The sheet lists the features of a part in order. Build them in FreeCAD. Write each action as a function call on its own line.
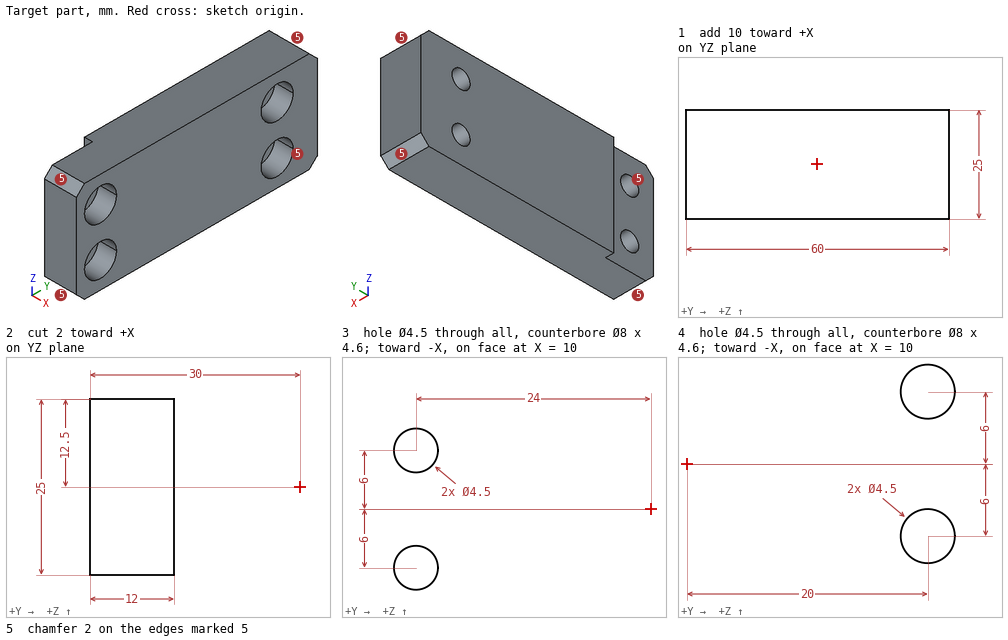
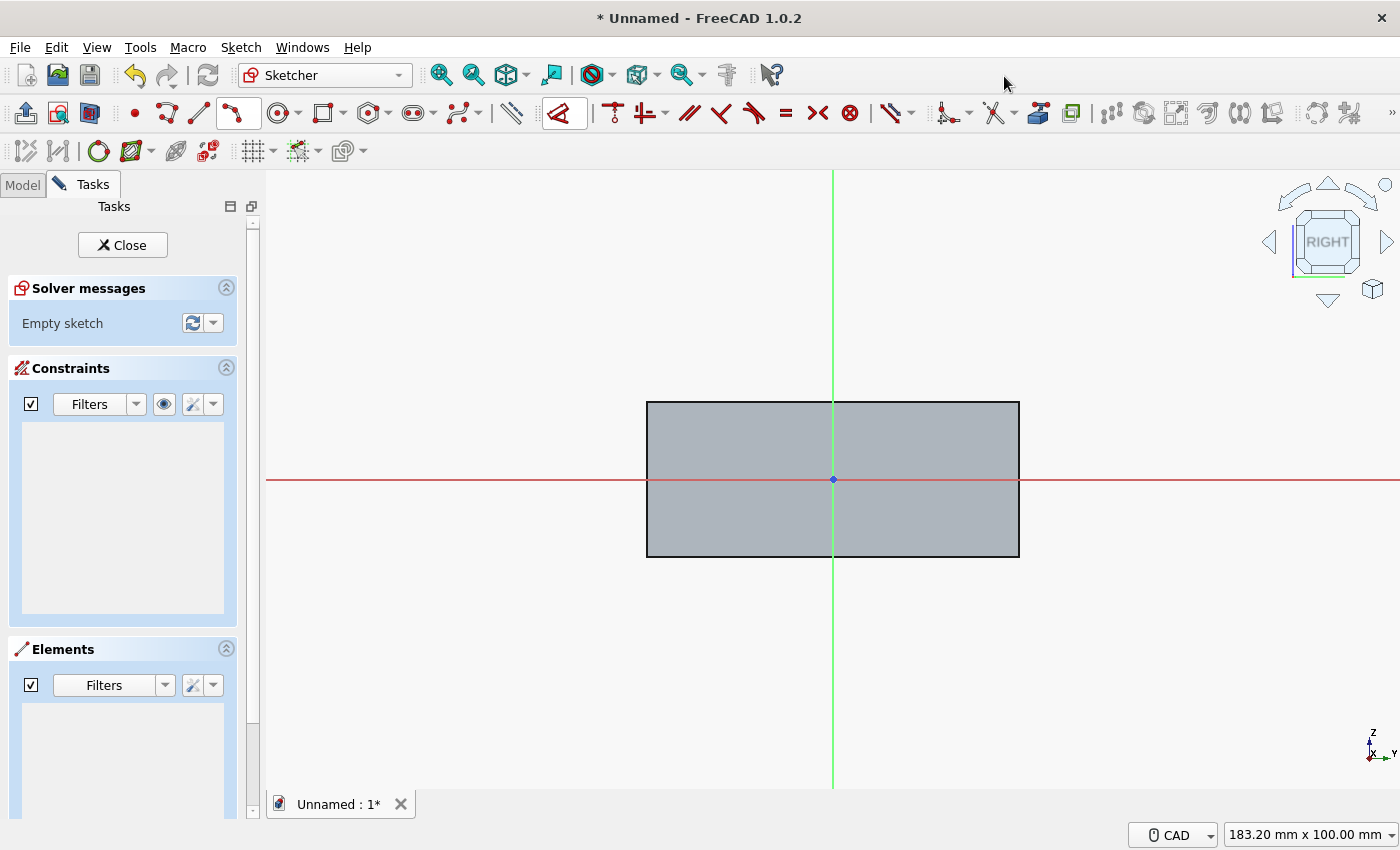
scroll(748, 480, up, 7)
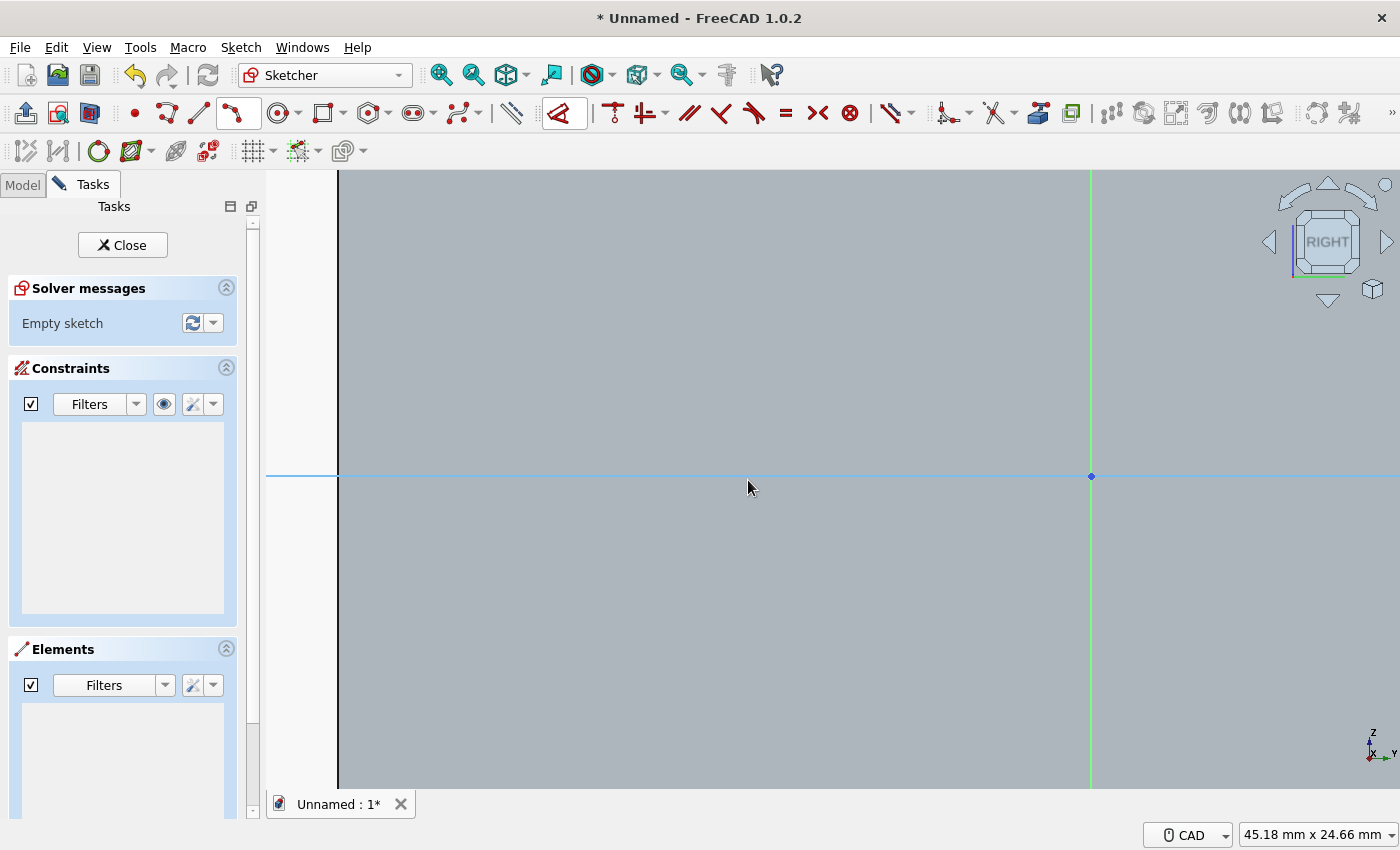
click(278, 114)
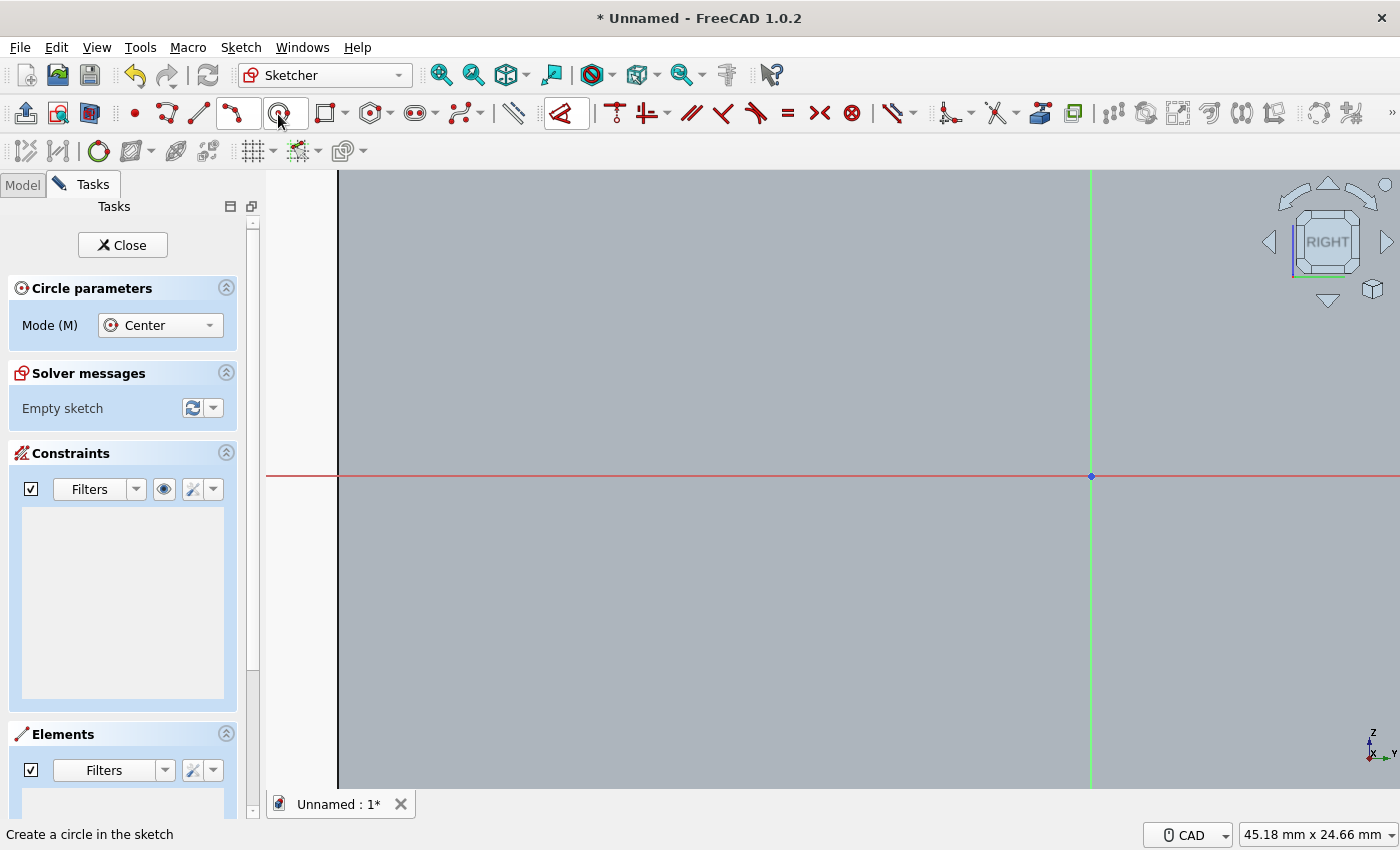
click(489, 326)
click(529, 286)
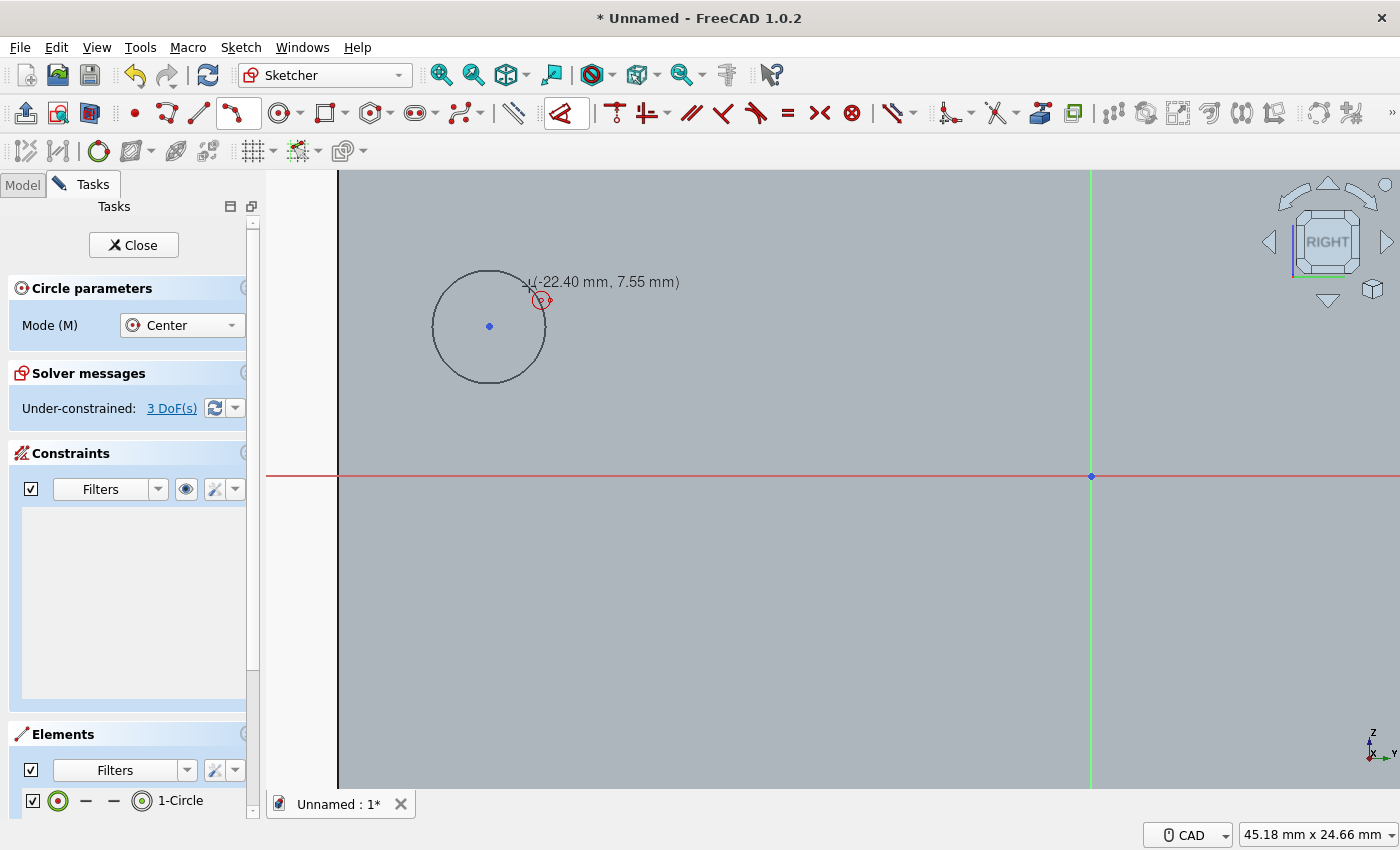
click(489, 627)
click(529, 587)
key(Escape)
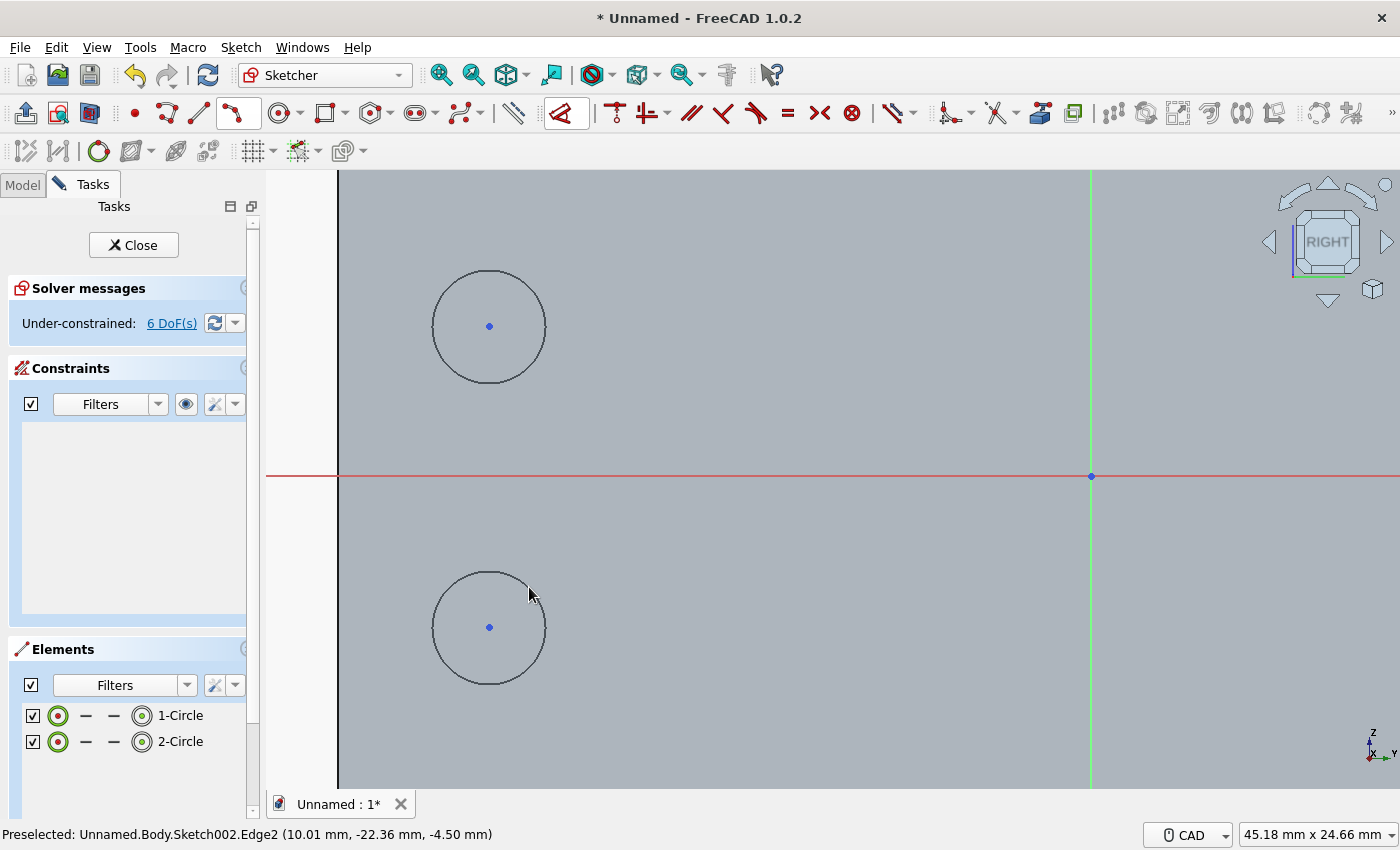
click(529, 287)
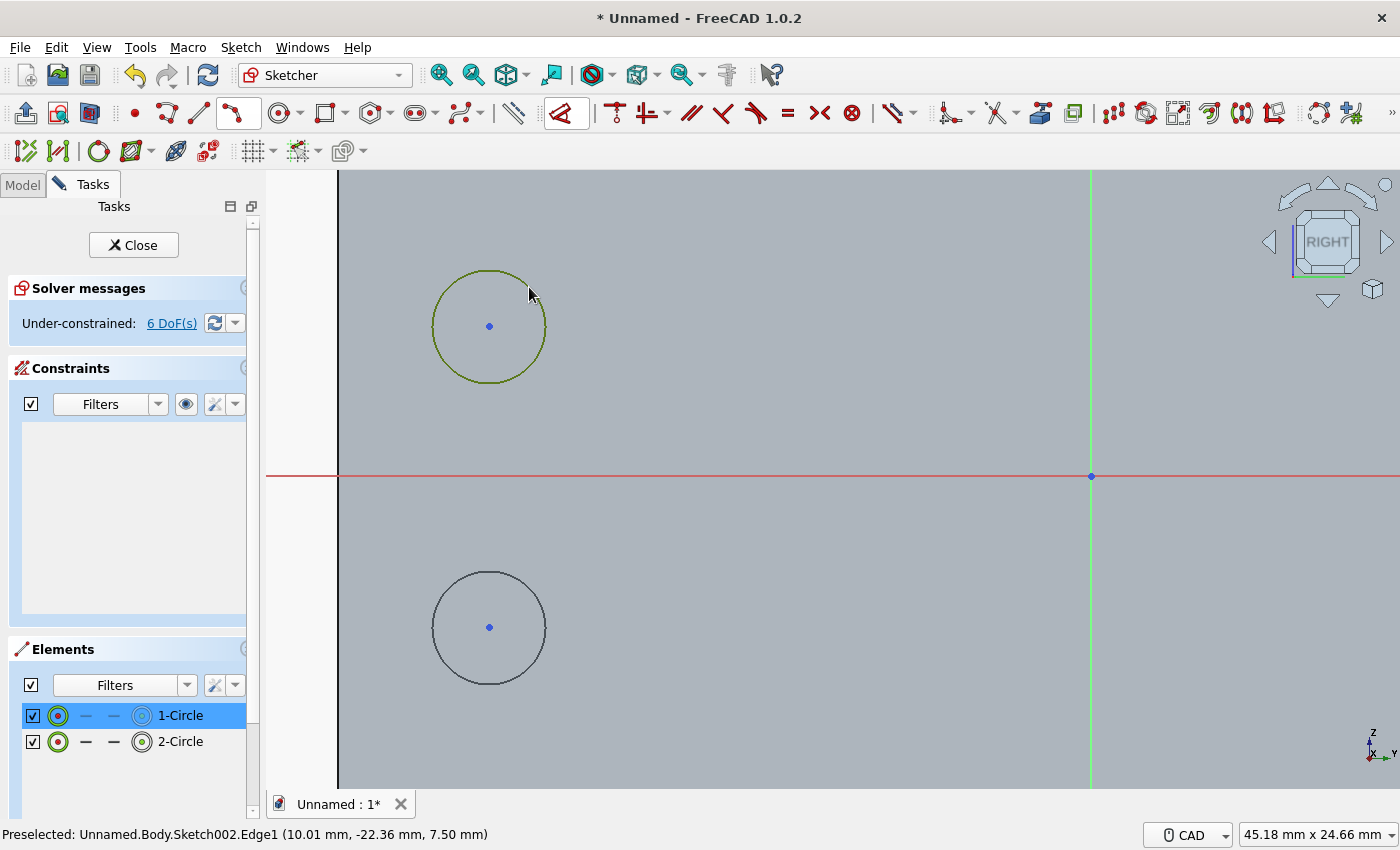
click(529, 588)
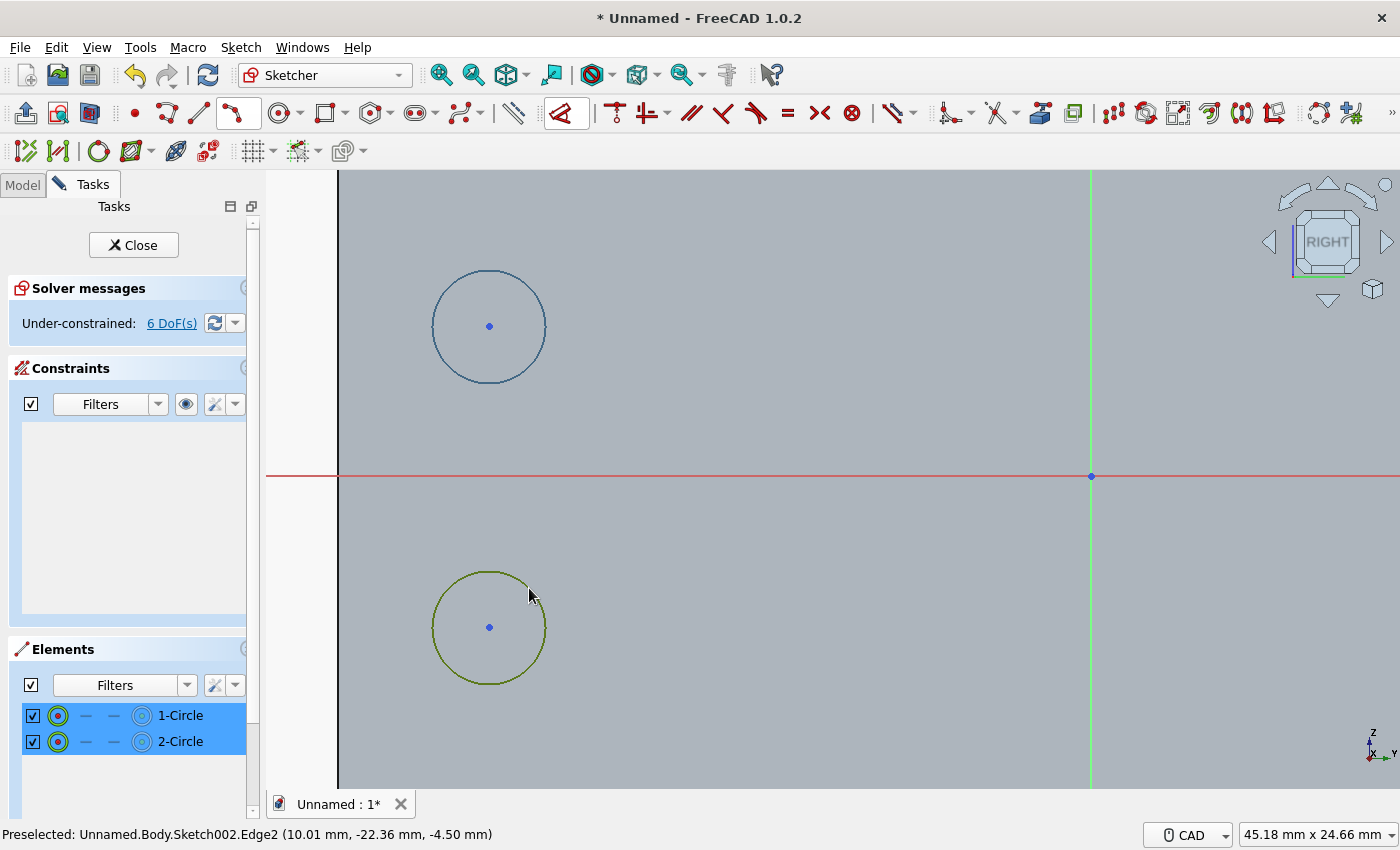
click(788, 114)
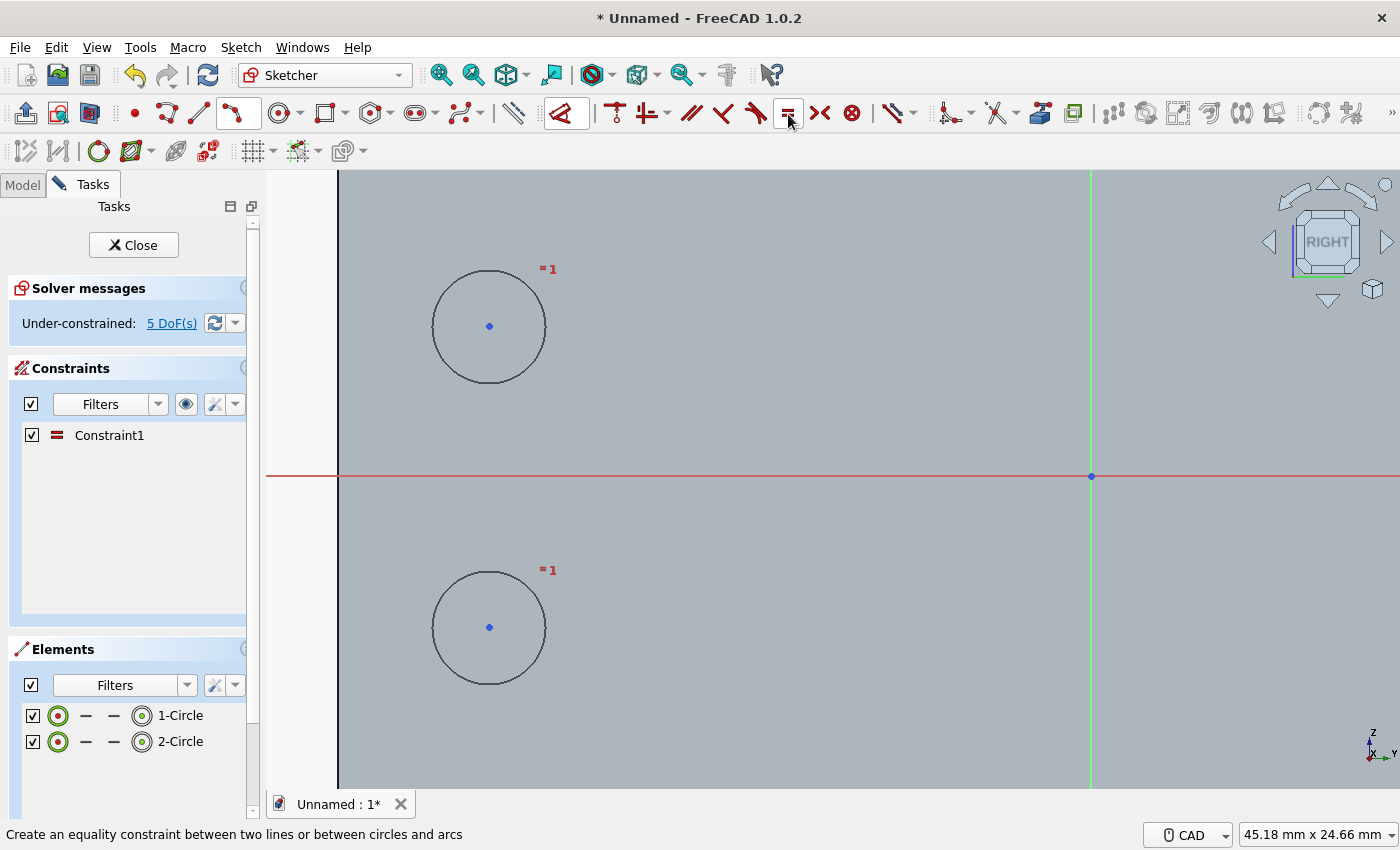
click(489, 327)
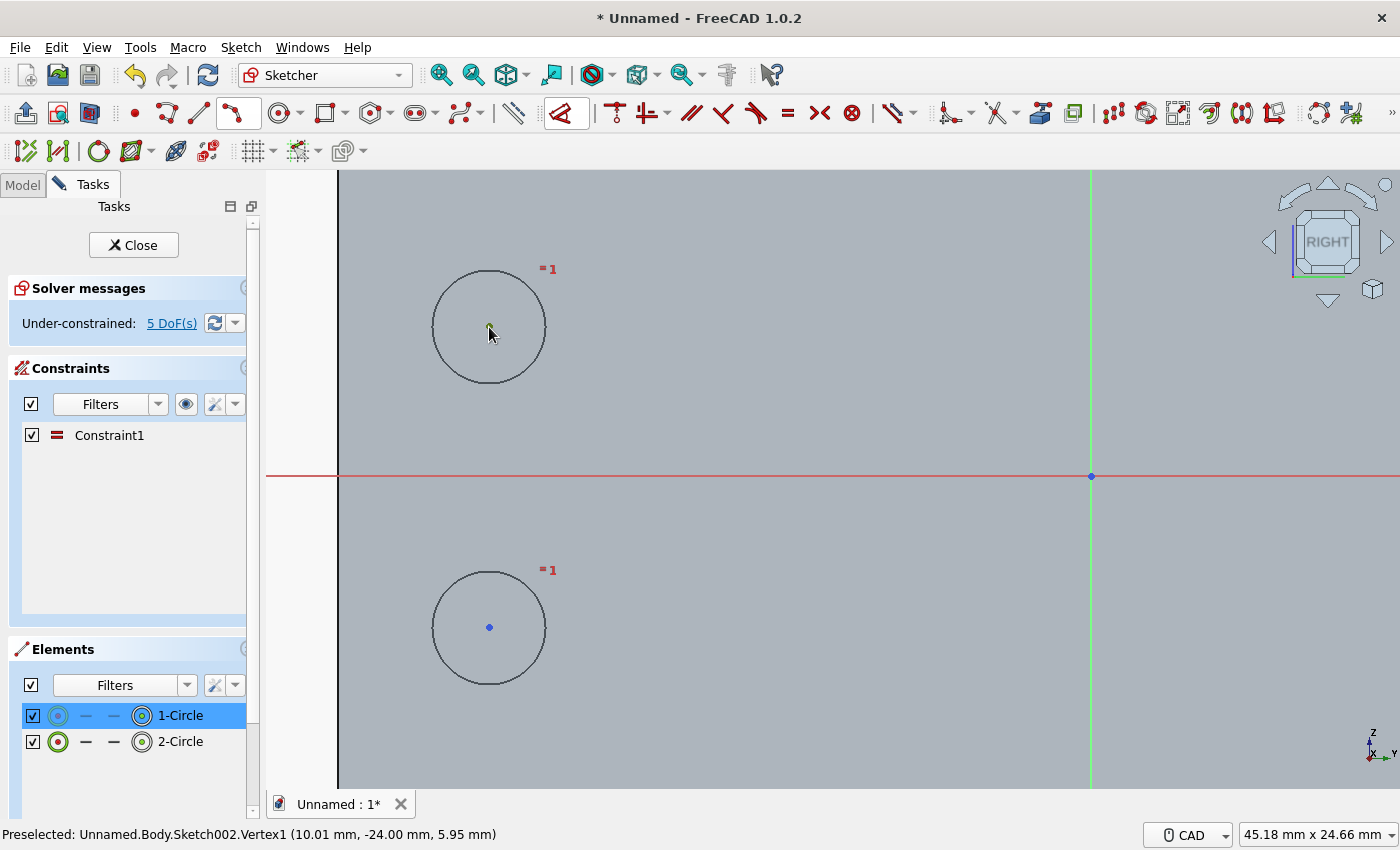
click(489, 628)